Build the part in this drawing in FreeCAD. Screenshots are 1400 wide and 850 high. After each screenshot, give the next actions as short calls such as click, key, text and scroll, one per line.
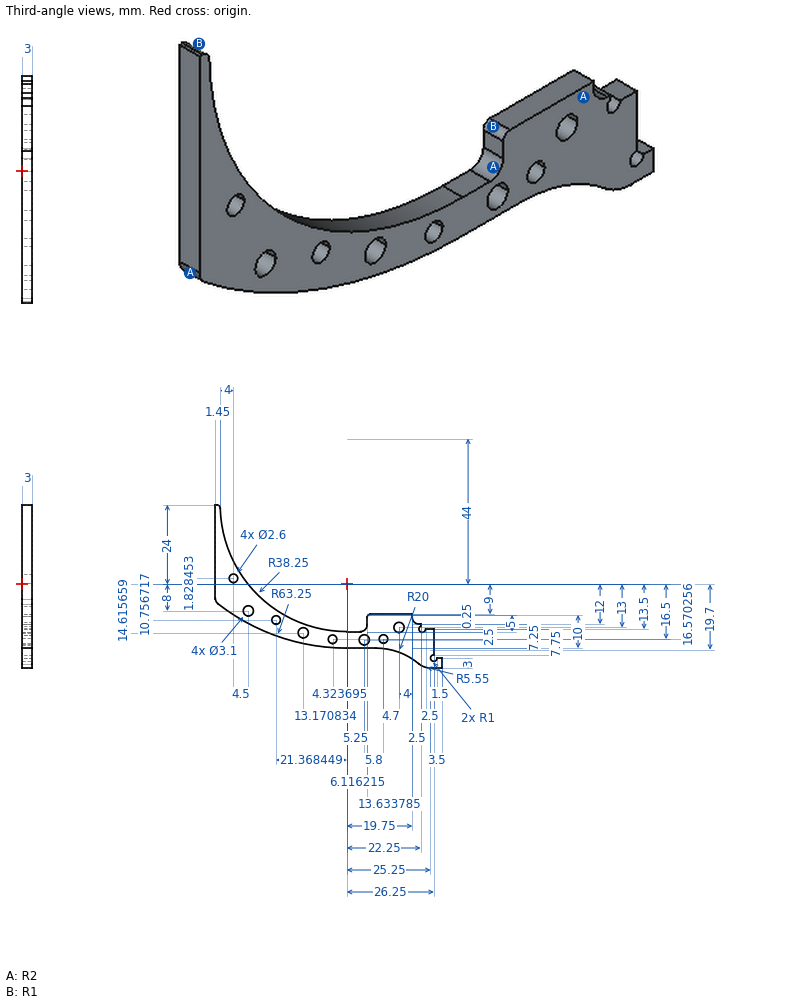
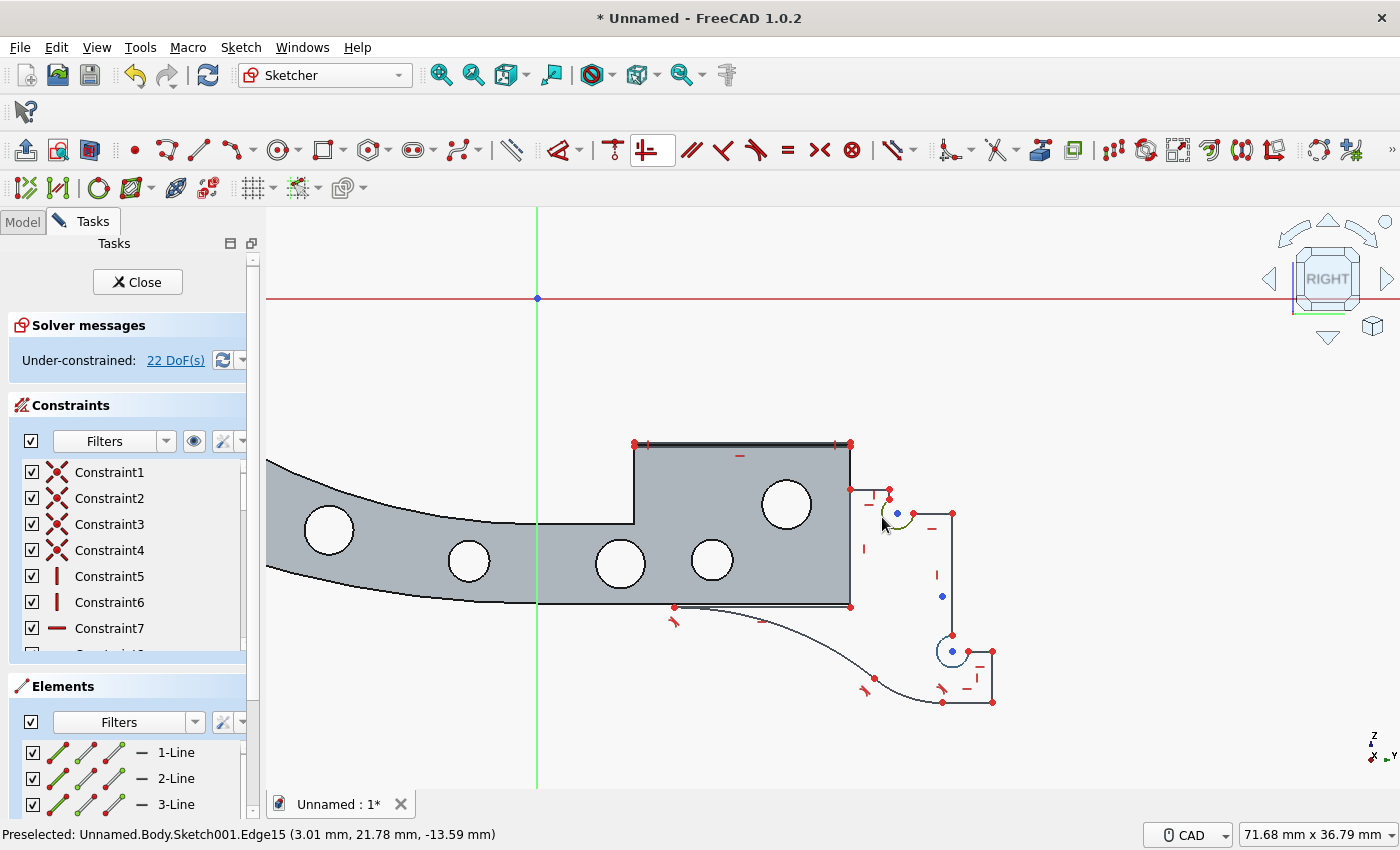
key(e)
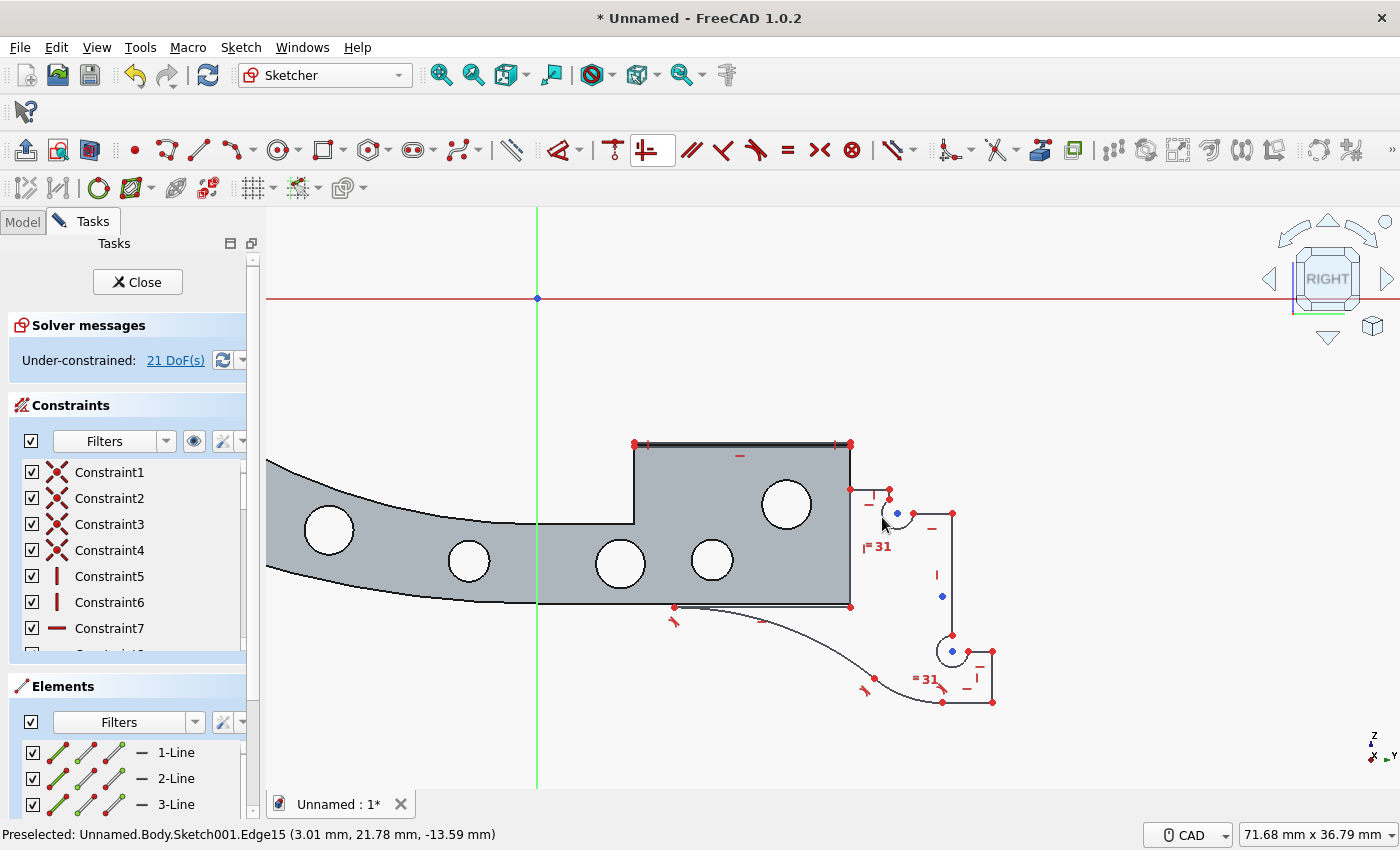
click(558, 150)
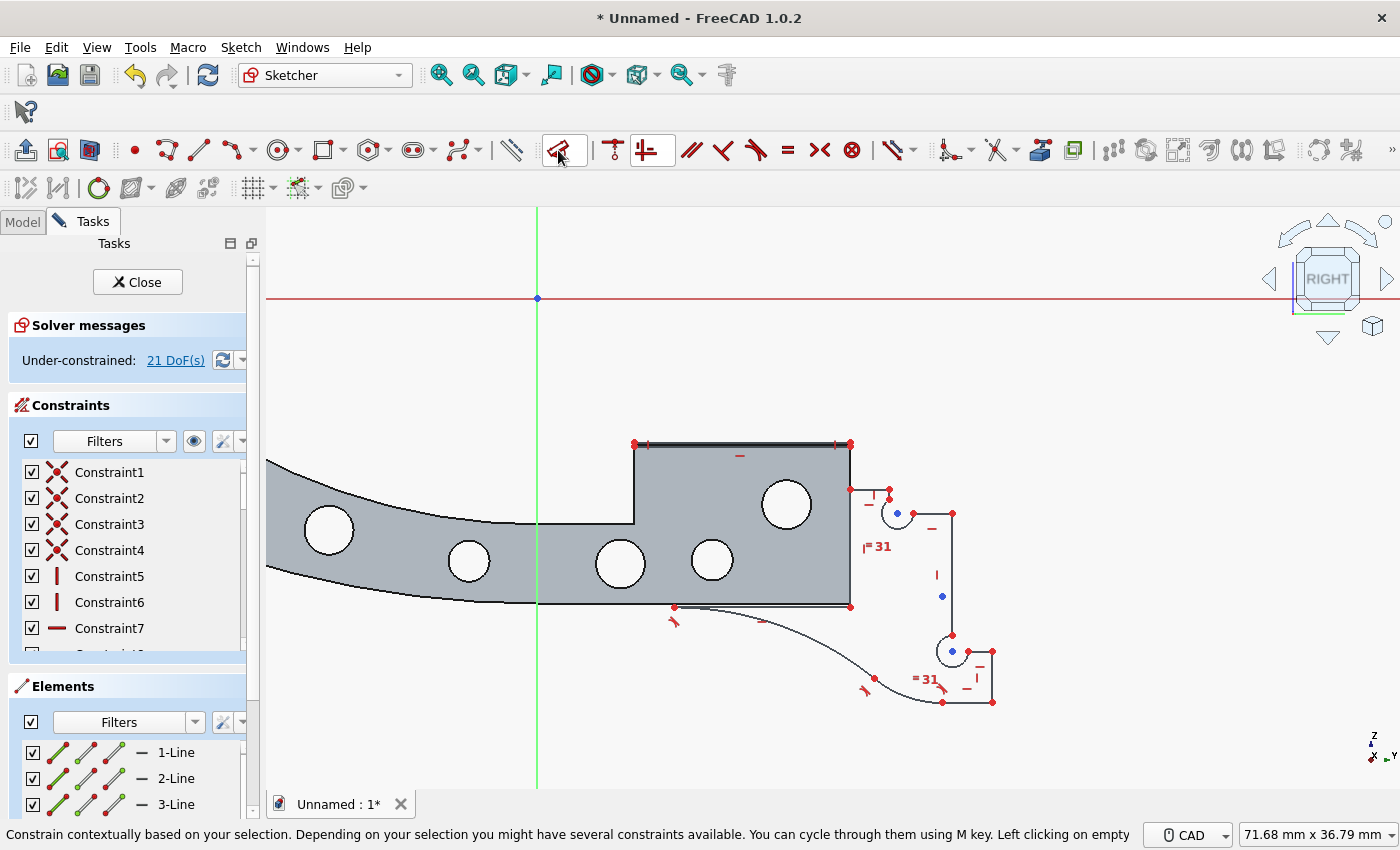
scroll(937, 649, up, 5)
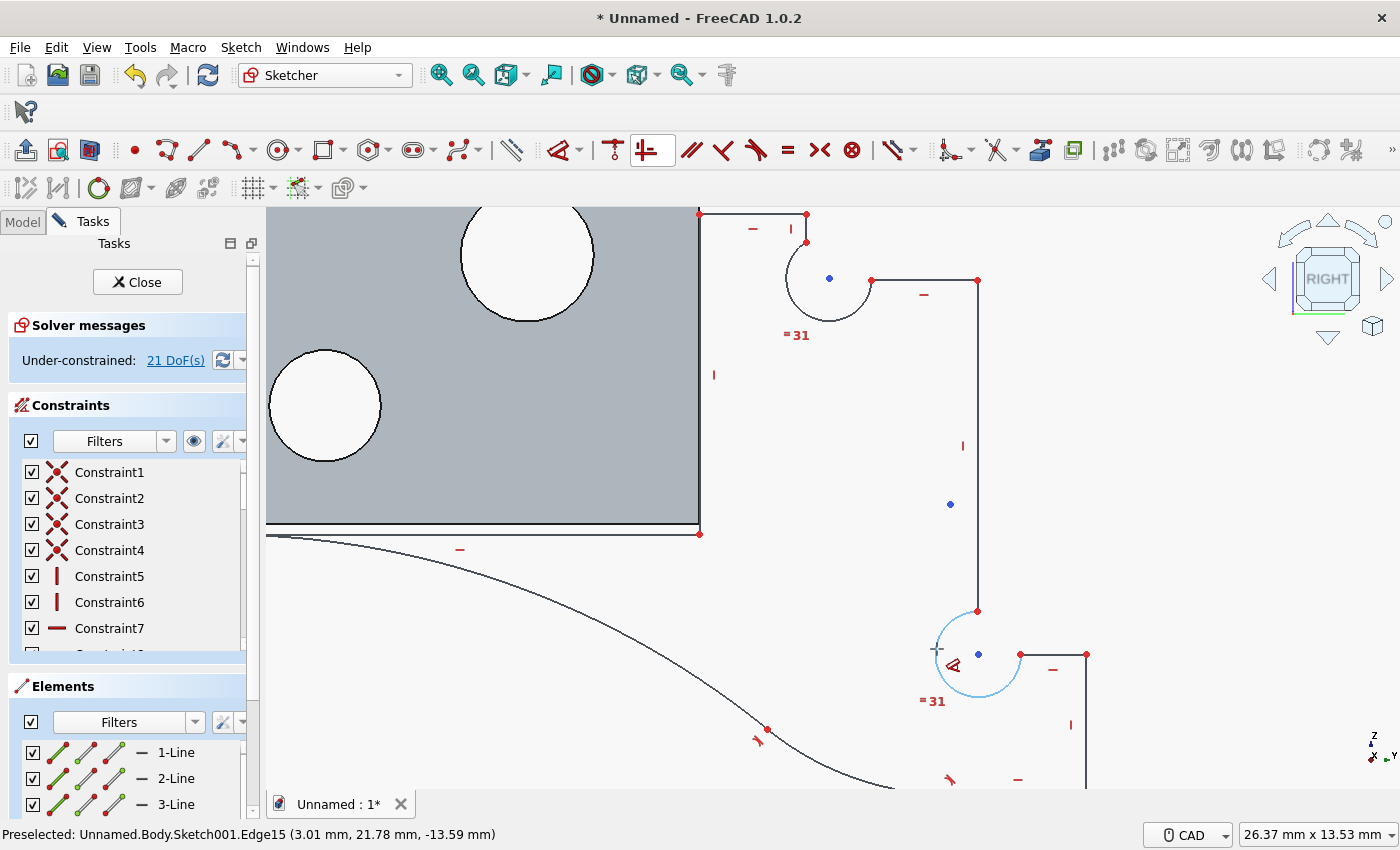
click(936, 648)
click(904, 643)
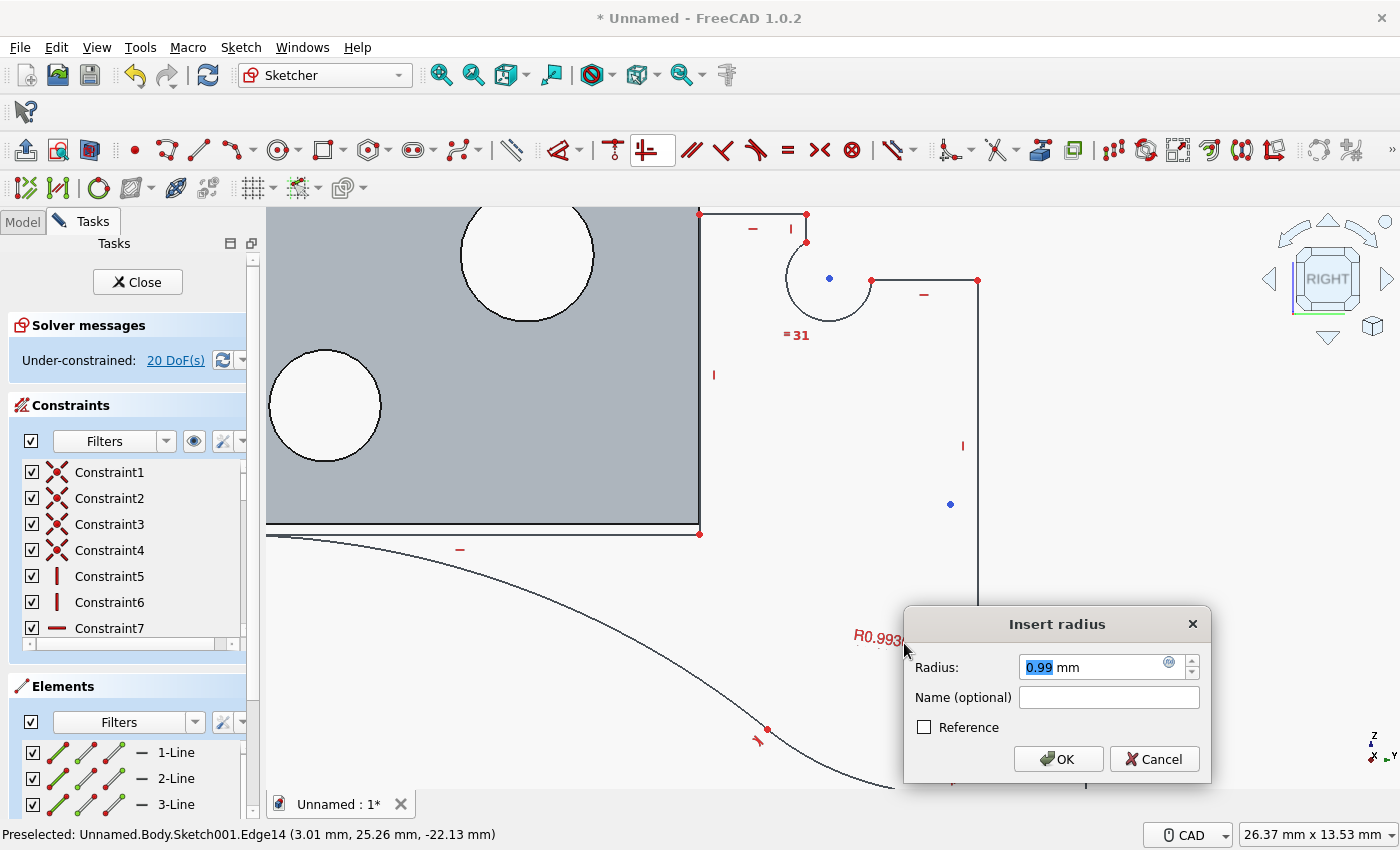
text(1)
key(Return)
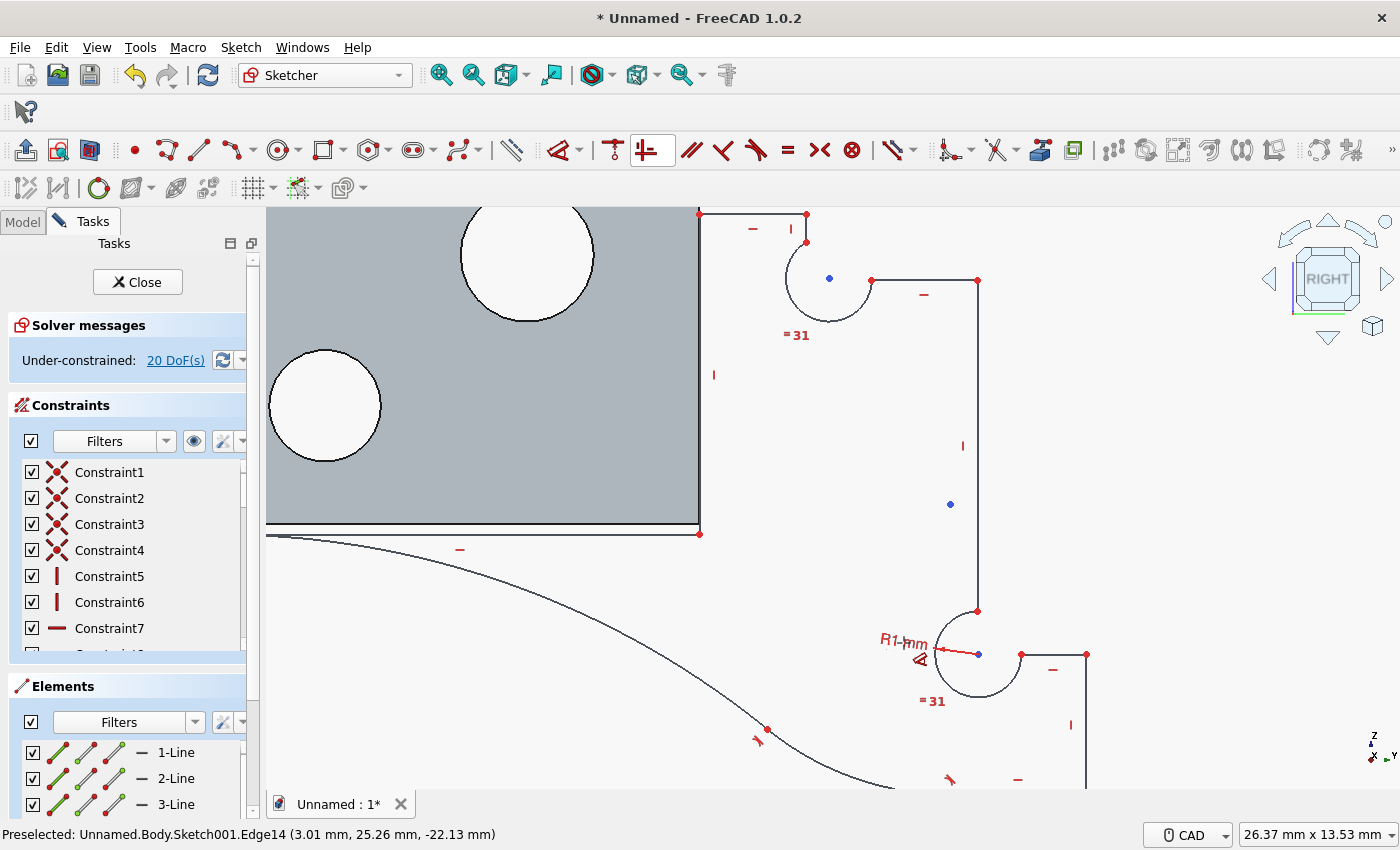
click(619, 632)
click(634, 604)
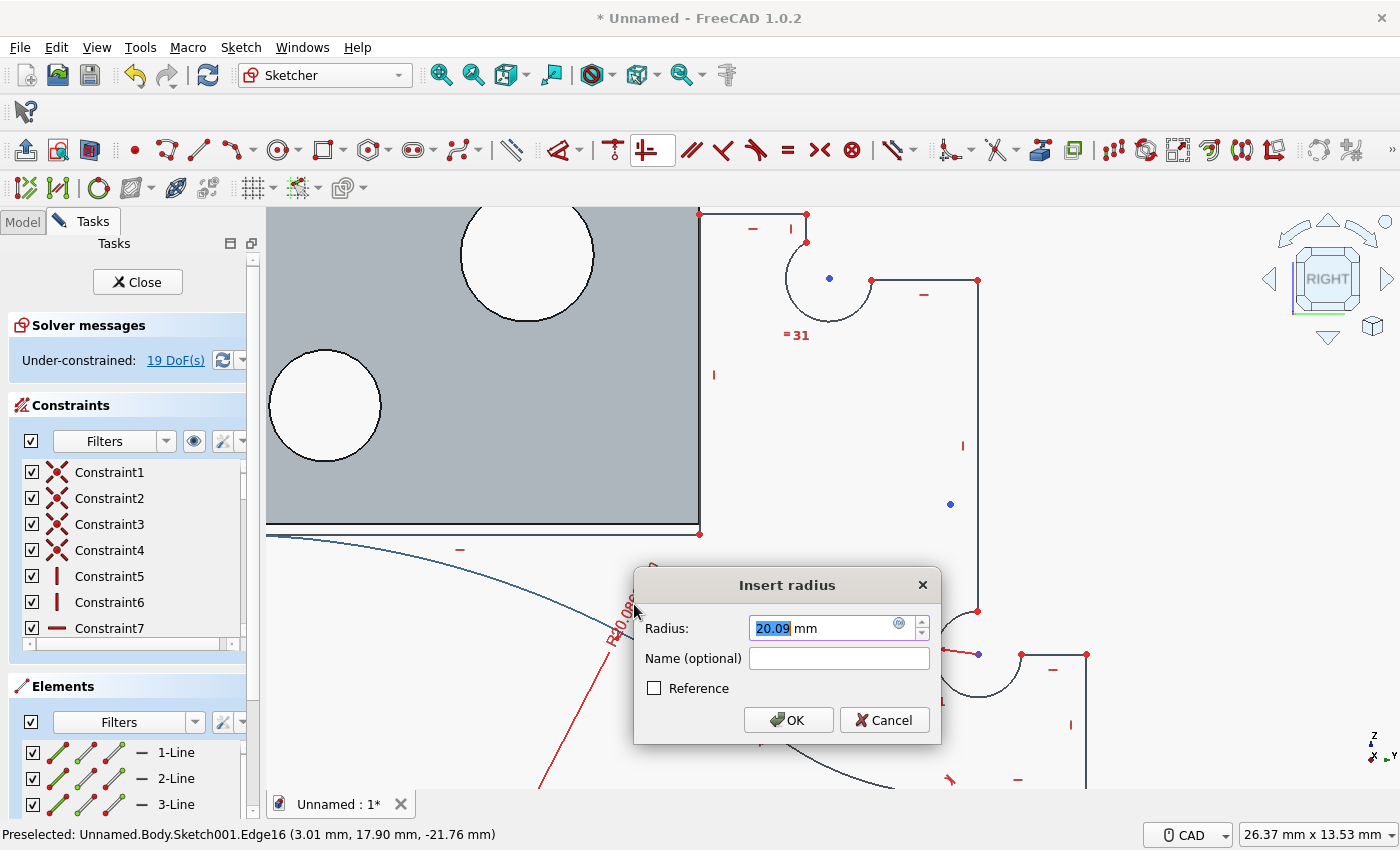
text(20)
key(Return)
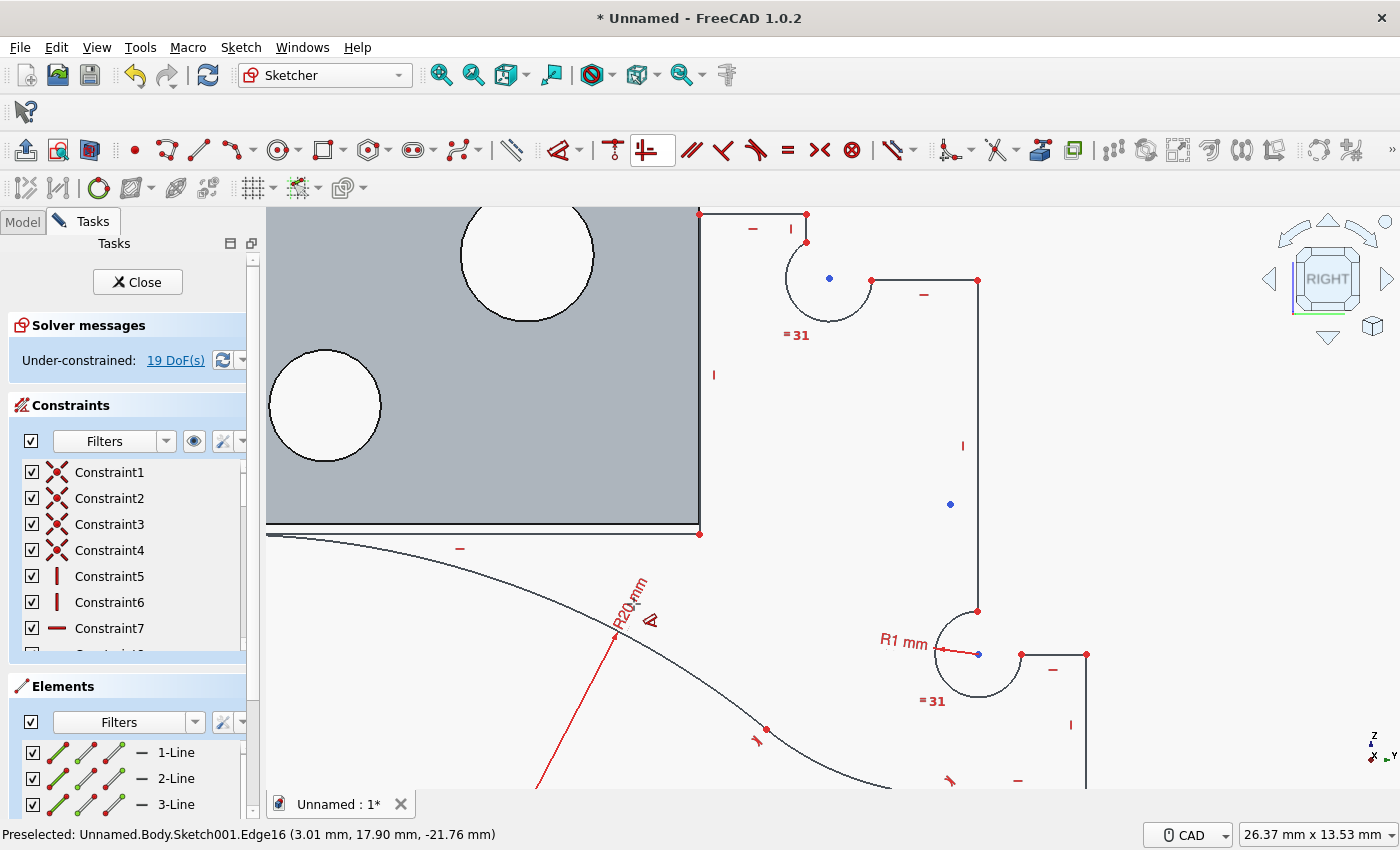
click(799, 752)
click(629, 512)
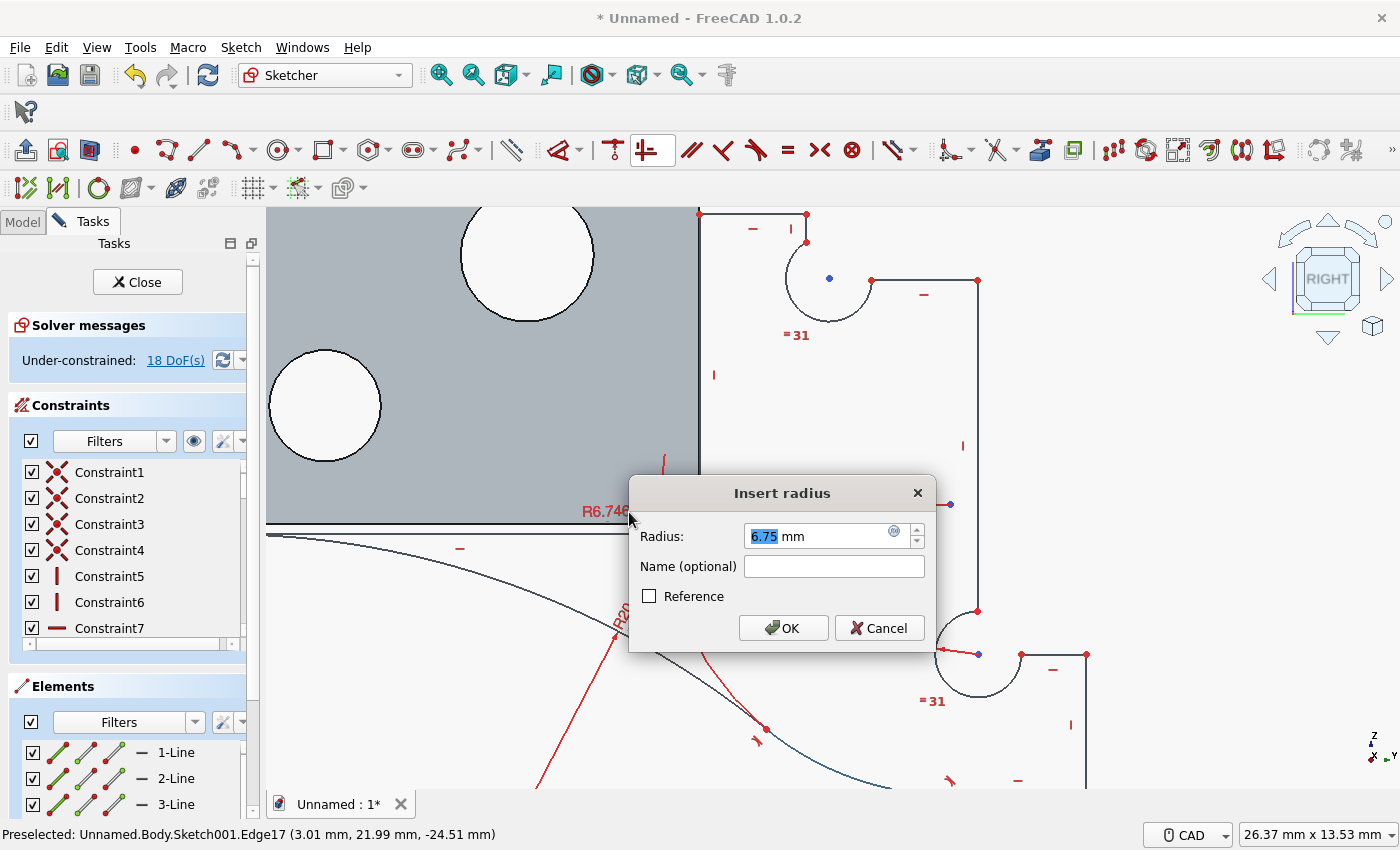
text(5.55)
key(Return)